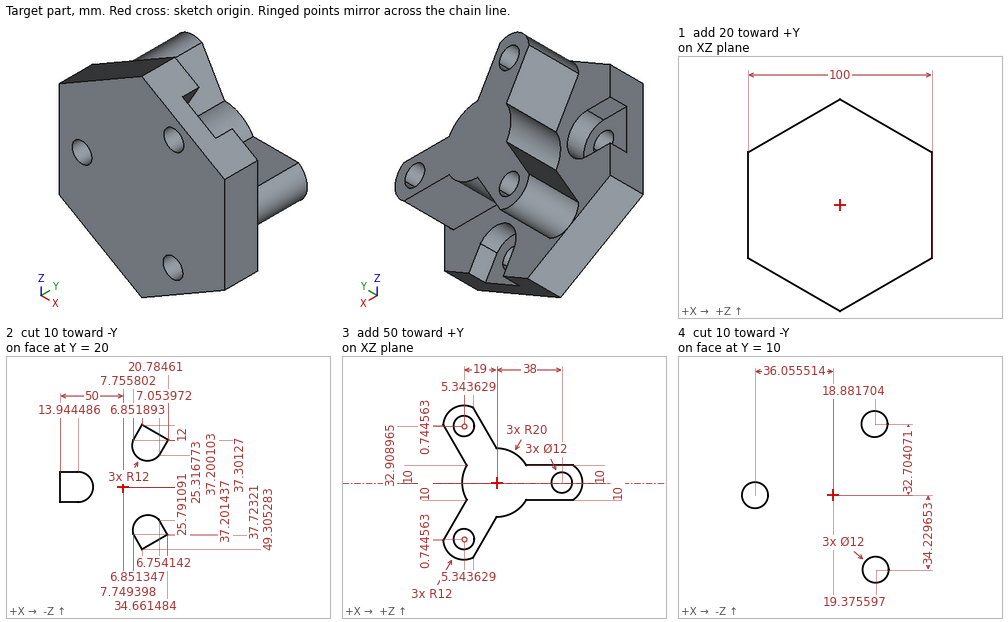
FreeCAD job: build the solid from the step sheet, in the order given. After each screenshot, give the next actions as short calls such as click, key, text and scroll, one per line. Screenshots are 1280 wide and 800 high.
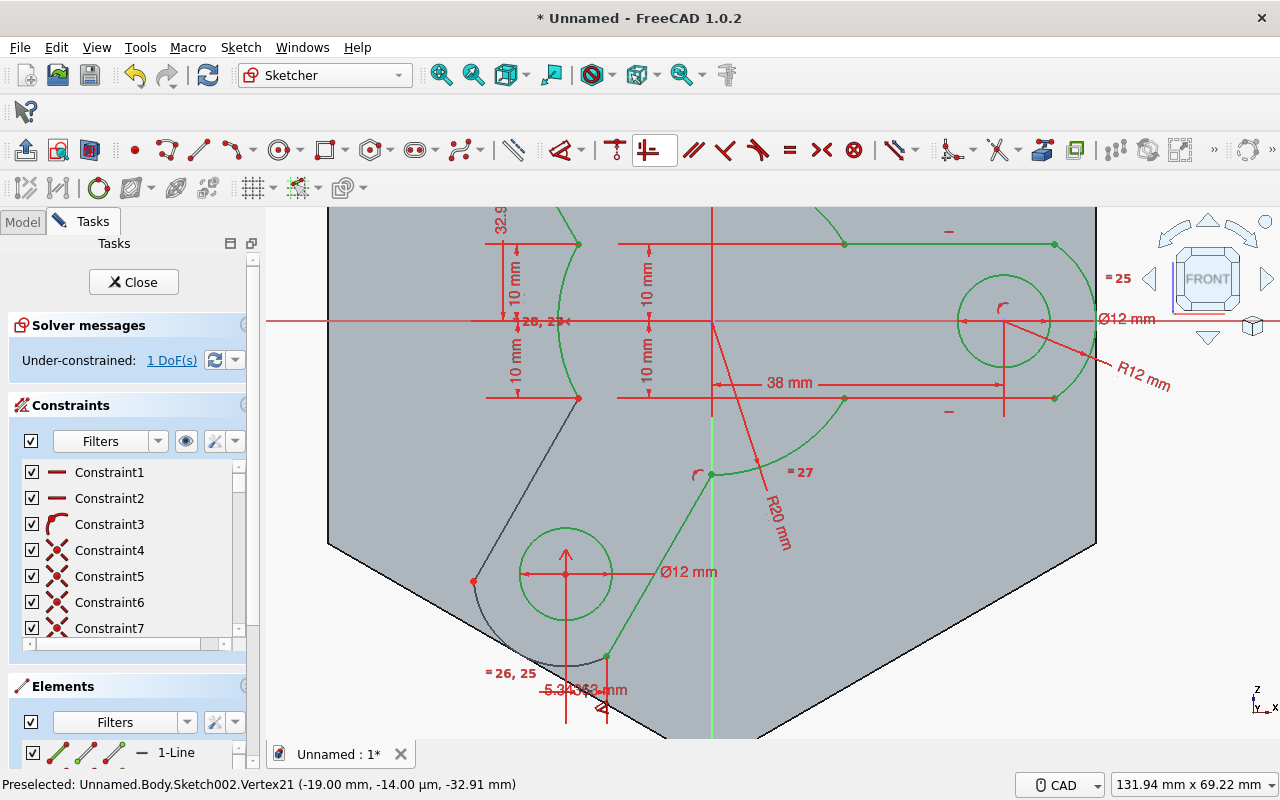
scroll(474, 582, up, 10)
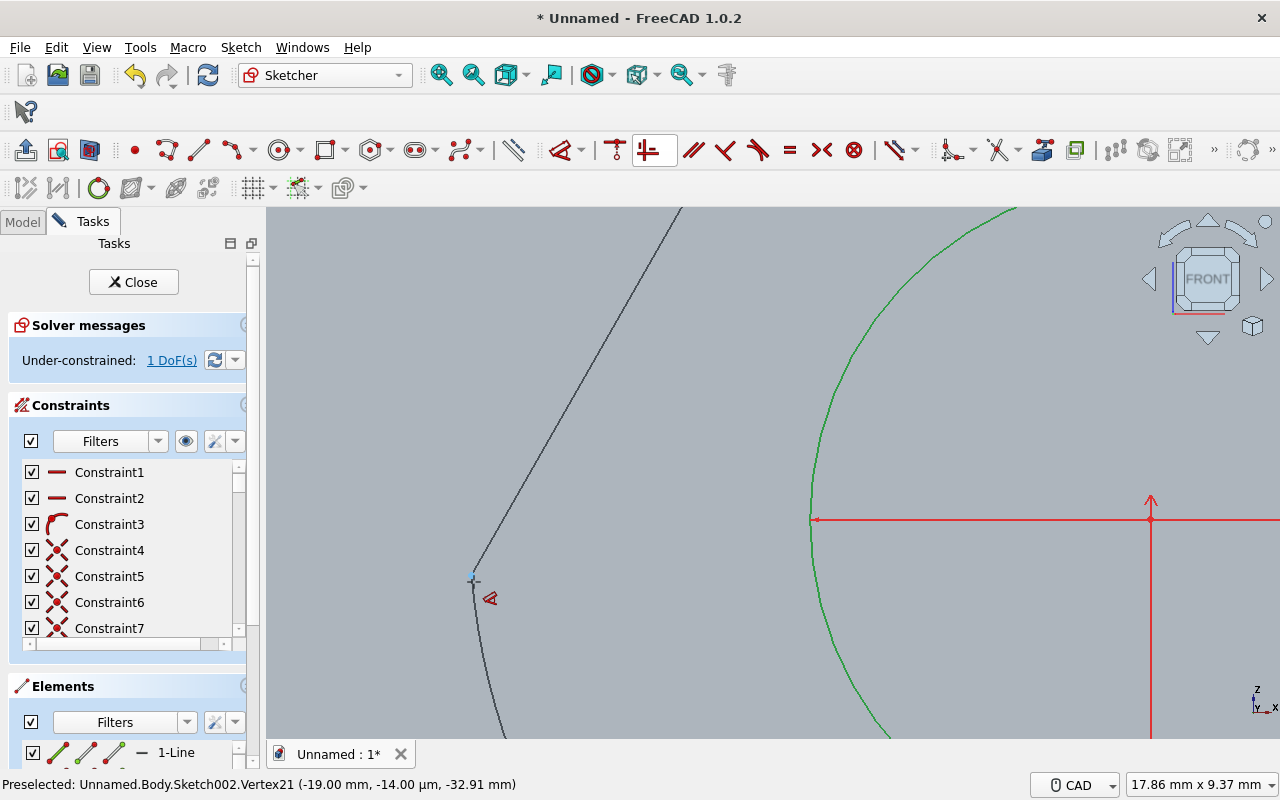
click(472, 575)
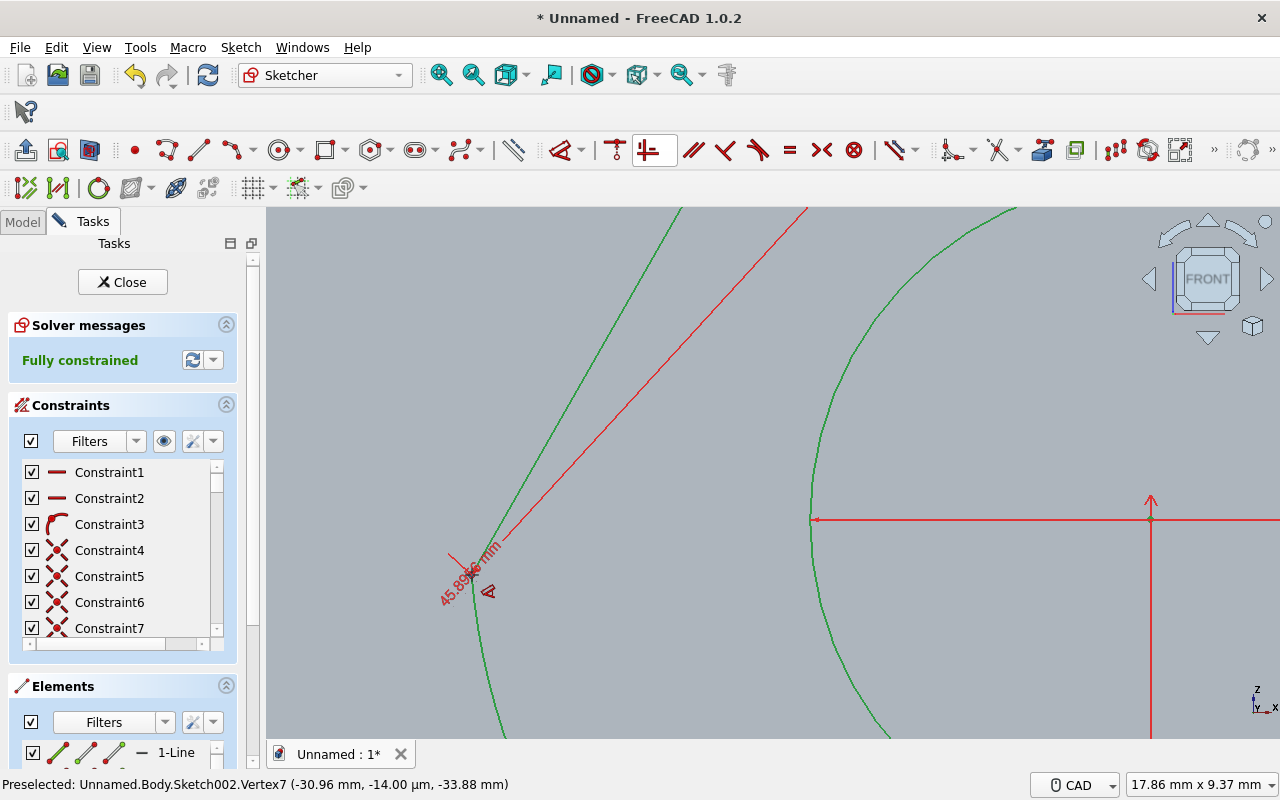
scroll(539, 619, down, 13)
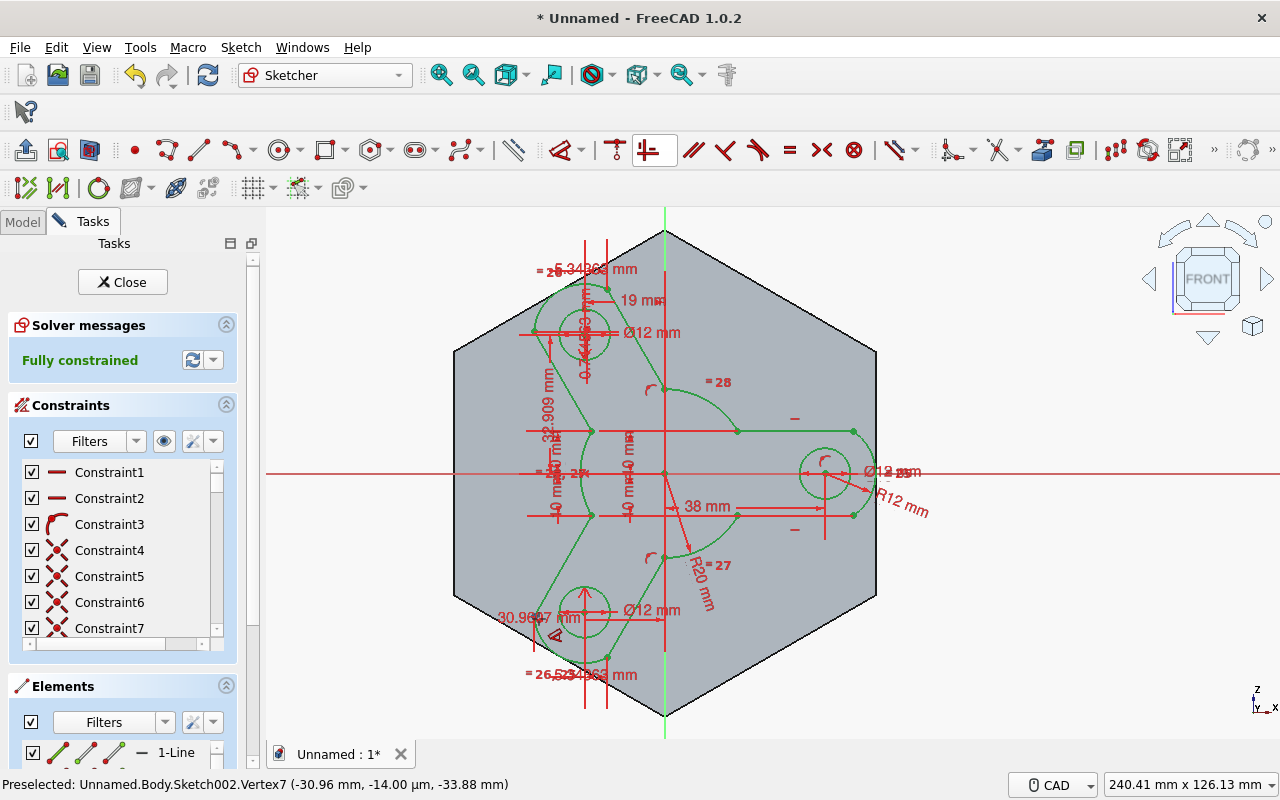
scroll(585, 612, up, 13)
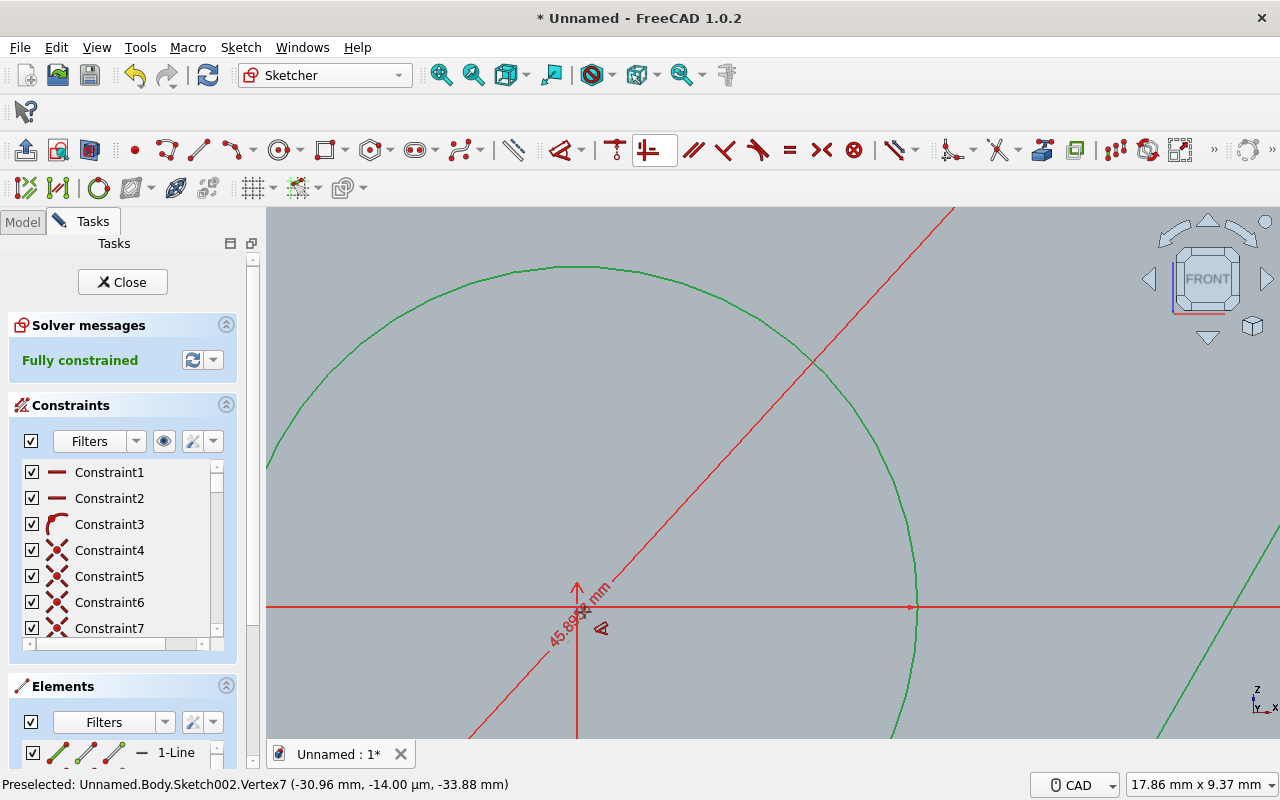
click(577, 607)
click(611, 635)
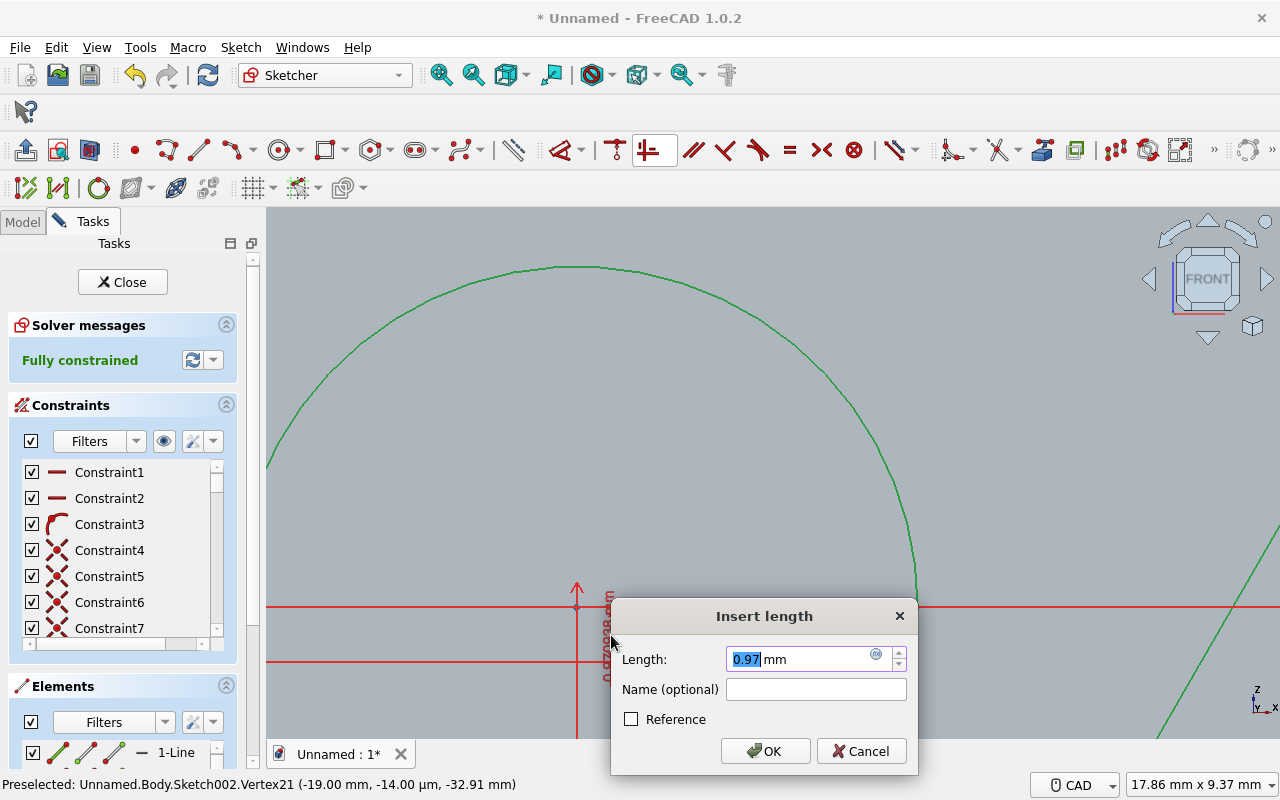
text(0.744563)
key(Return)
key(Escape)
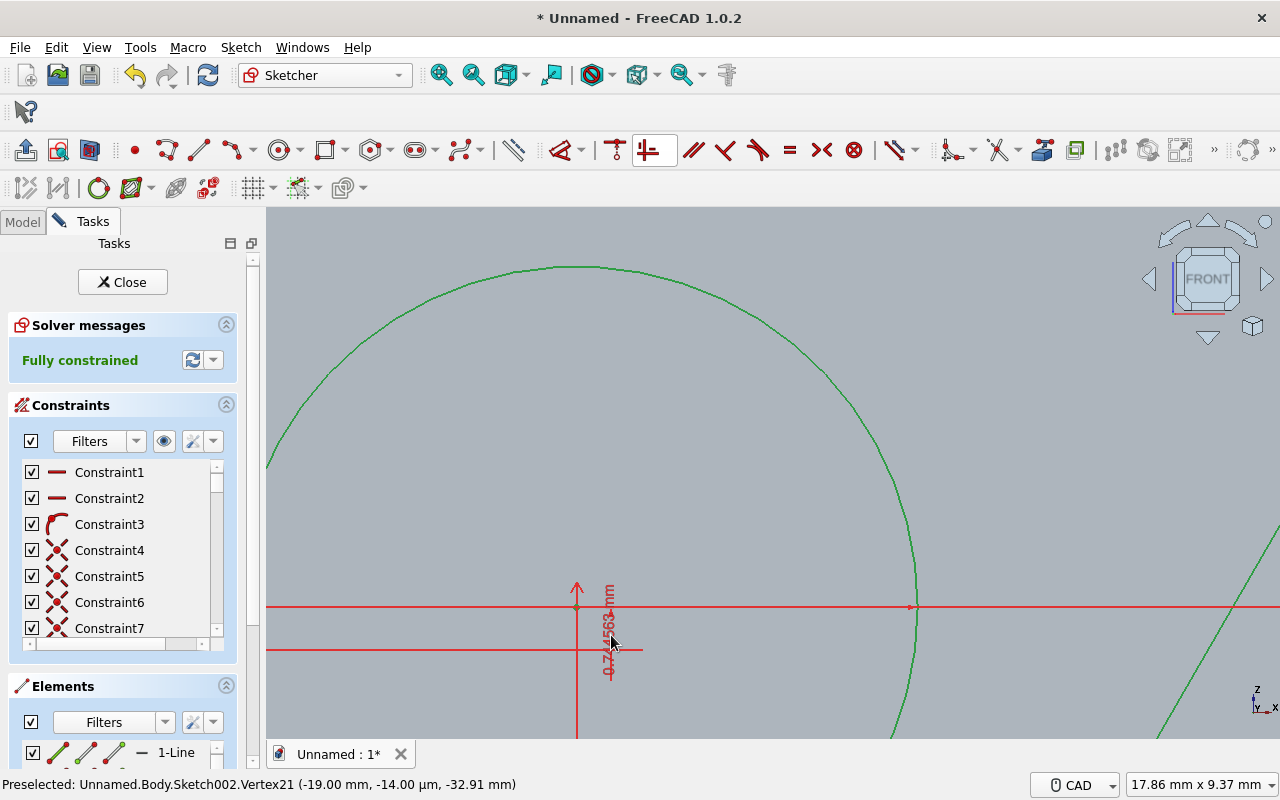
click(123, 282)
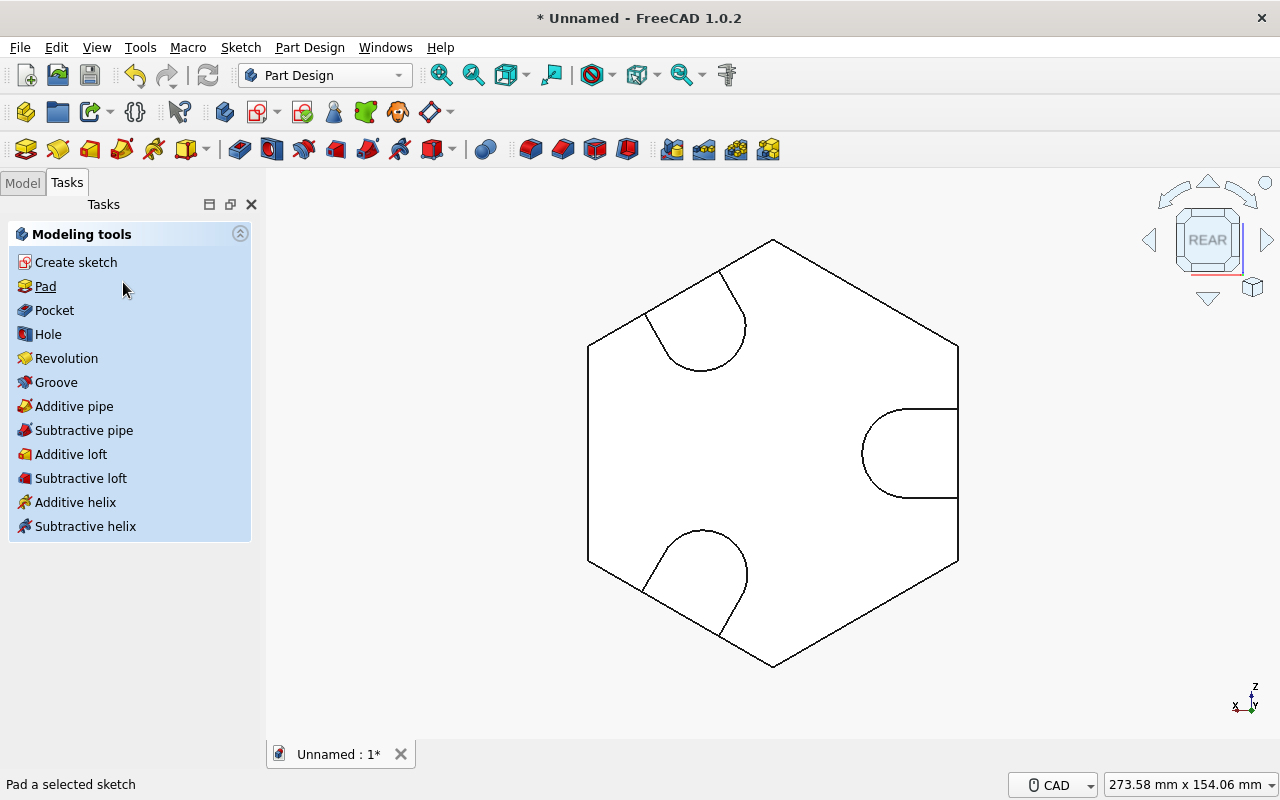
click(26, 150)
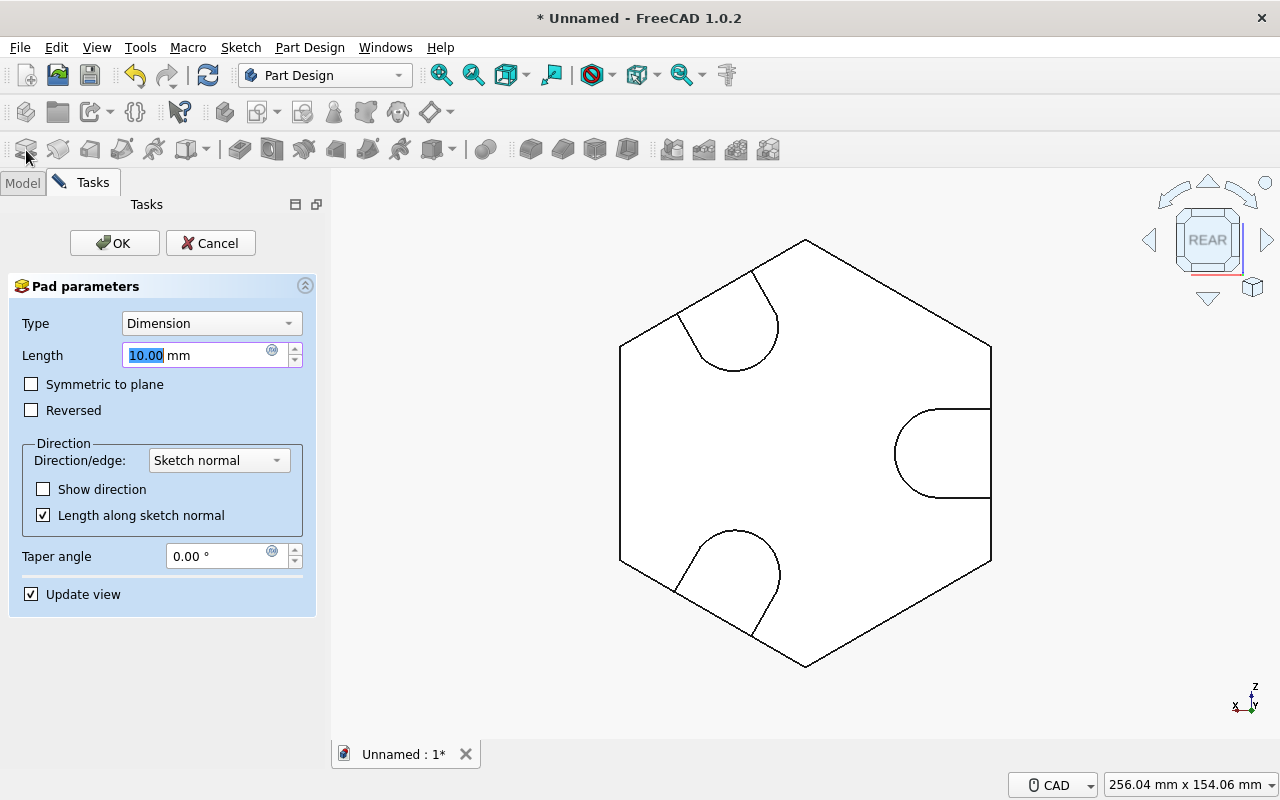
text(50)
key(Tab)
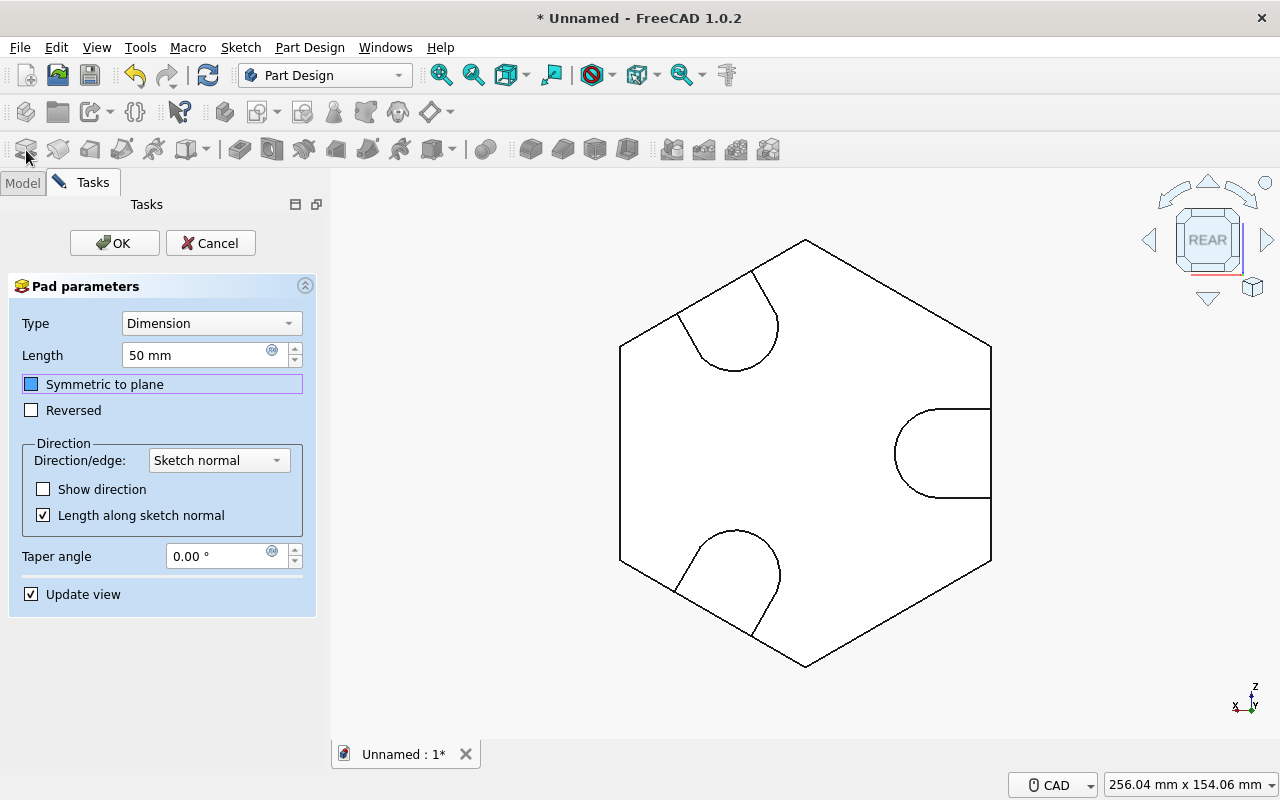
click(30, 410)